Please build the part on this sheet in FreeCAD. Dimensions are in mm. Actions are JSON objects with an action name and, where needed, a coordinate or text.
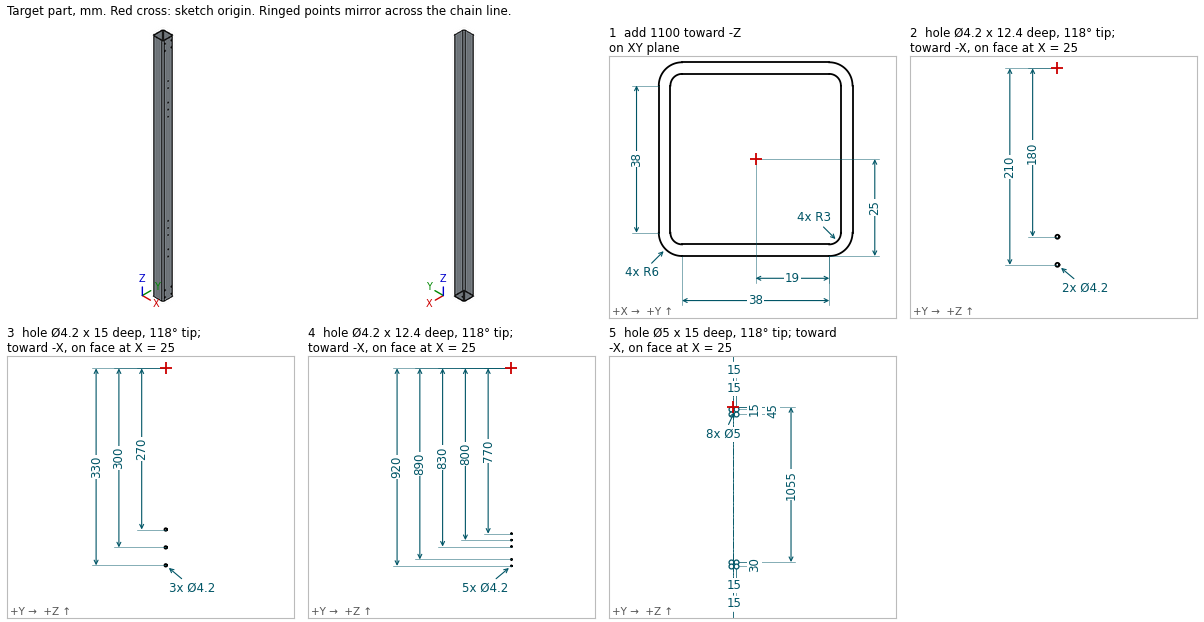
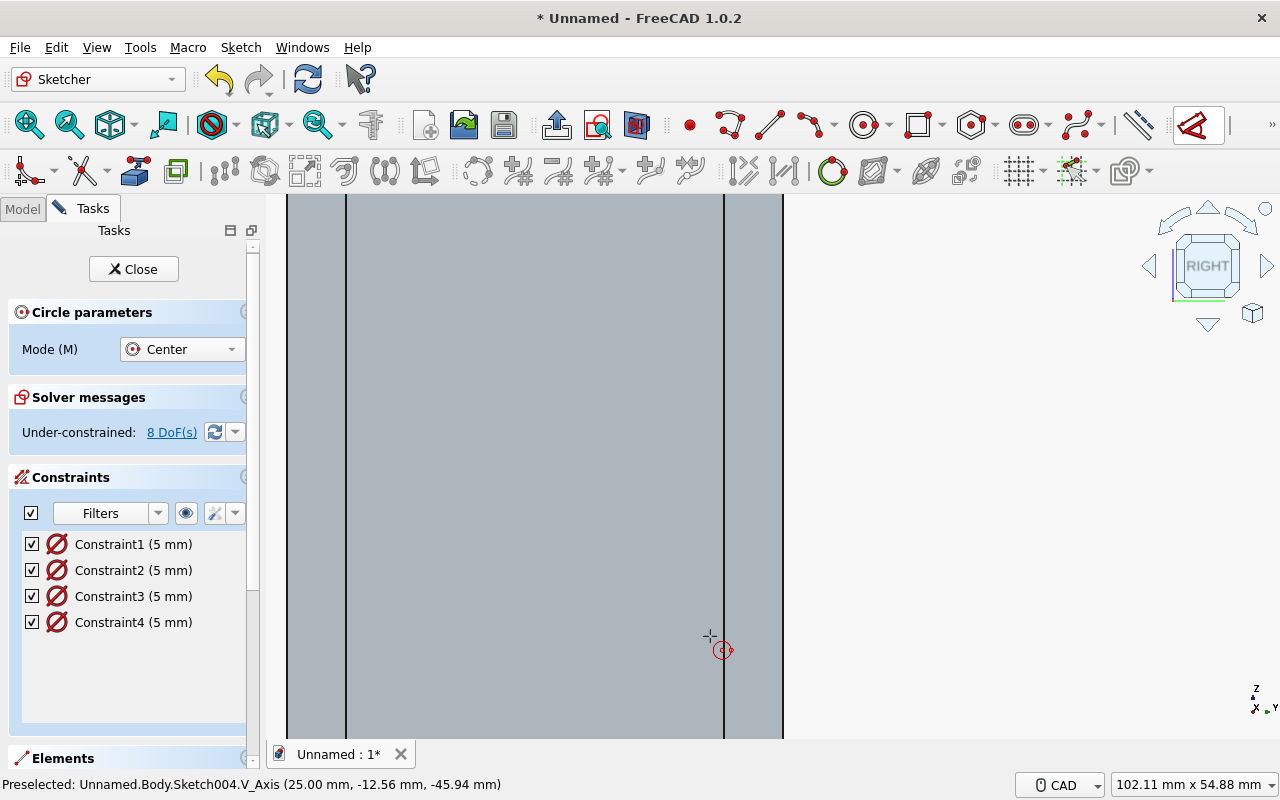
{"action": "scroll", "coordinate": [710, 637], "scroll_direction": "down", "scroll_amount": 17}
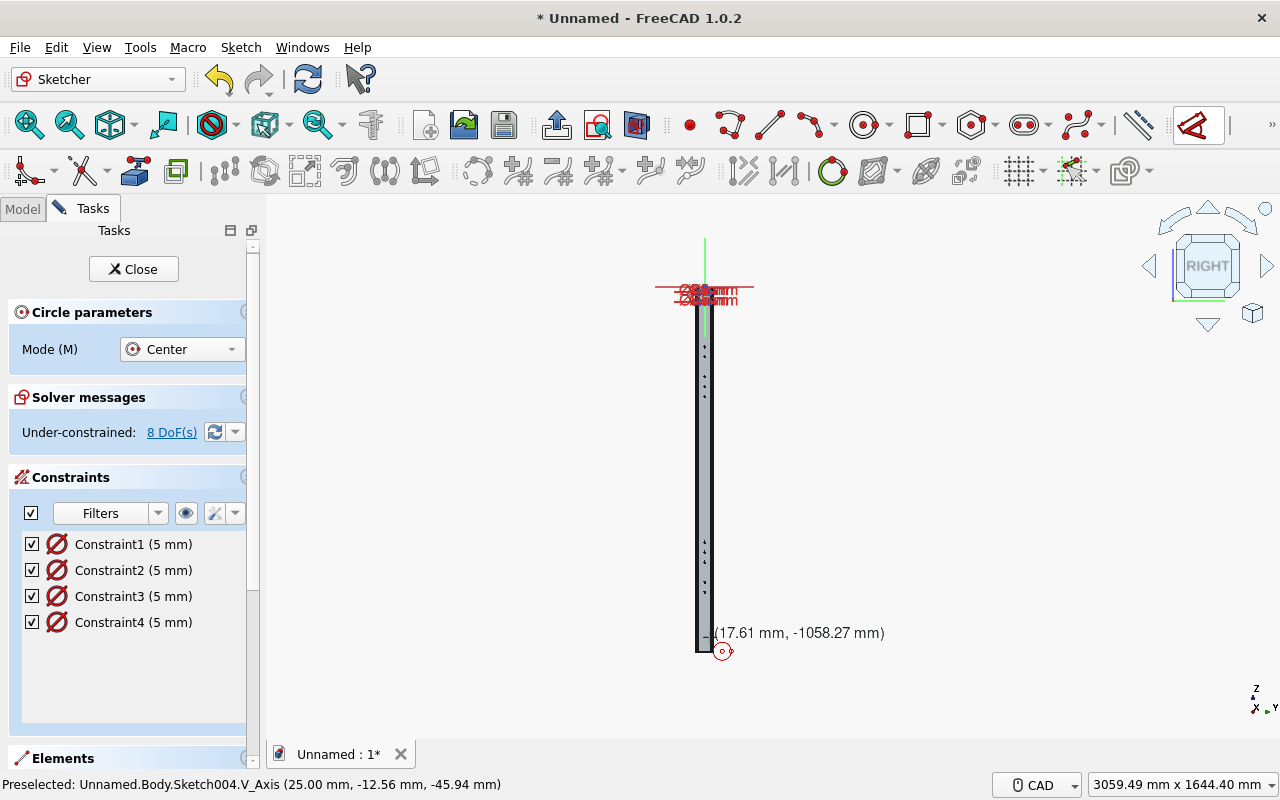
{"action": "scroll", "coordinate": [710, 637], "scroll_direction": "up", "scroll_amount": 6}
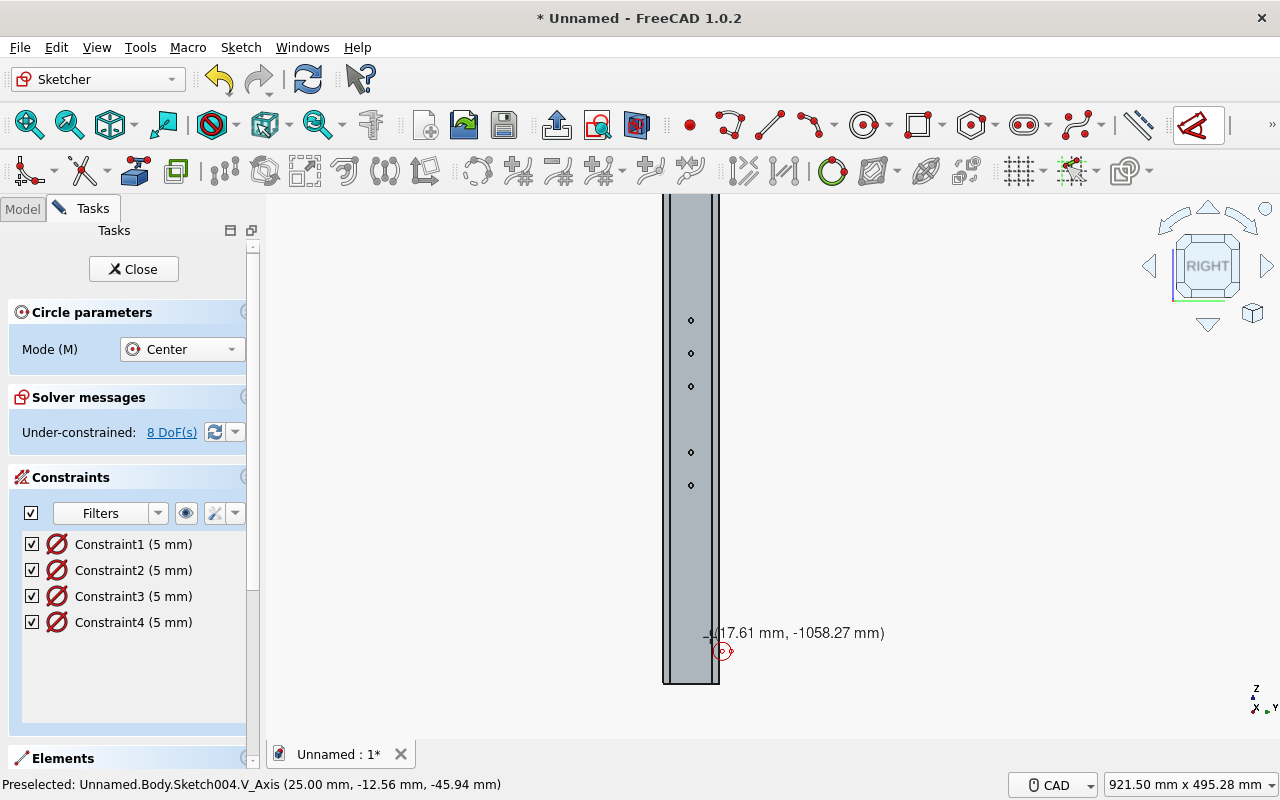
{"action": "left_click", "coordinate": [708, 634]}
{"action": "mouse_move", "coordinate": [709, 632]}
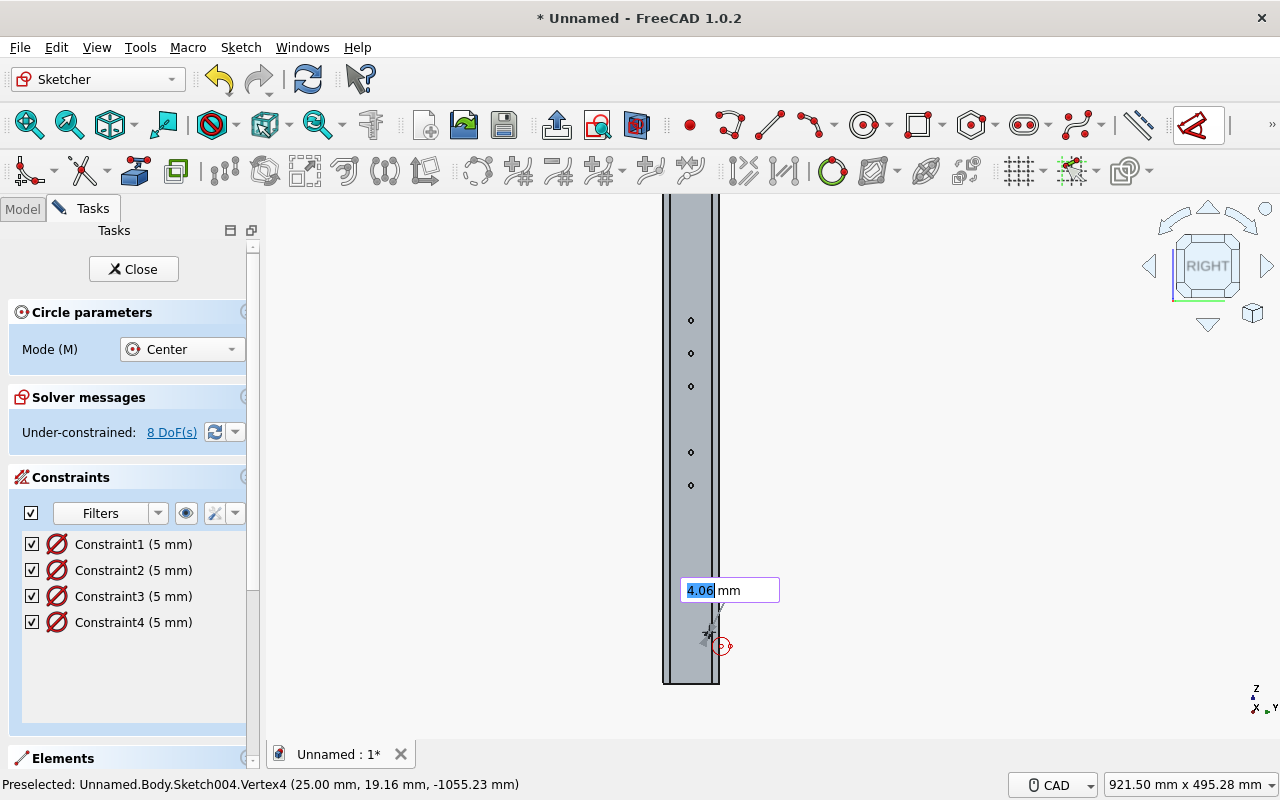
{"action": "type", "text": "5"}
{"action": "key", "text": "Return"}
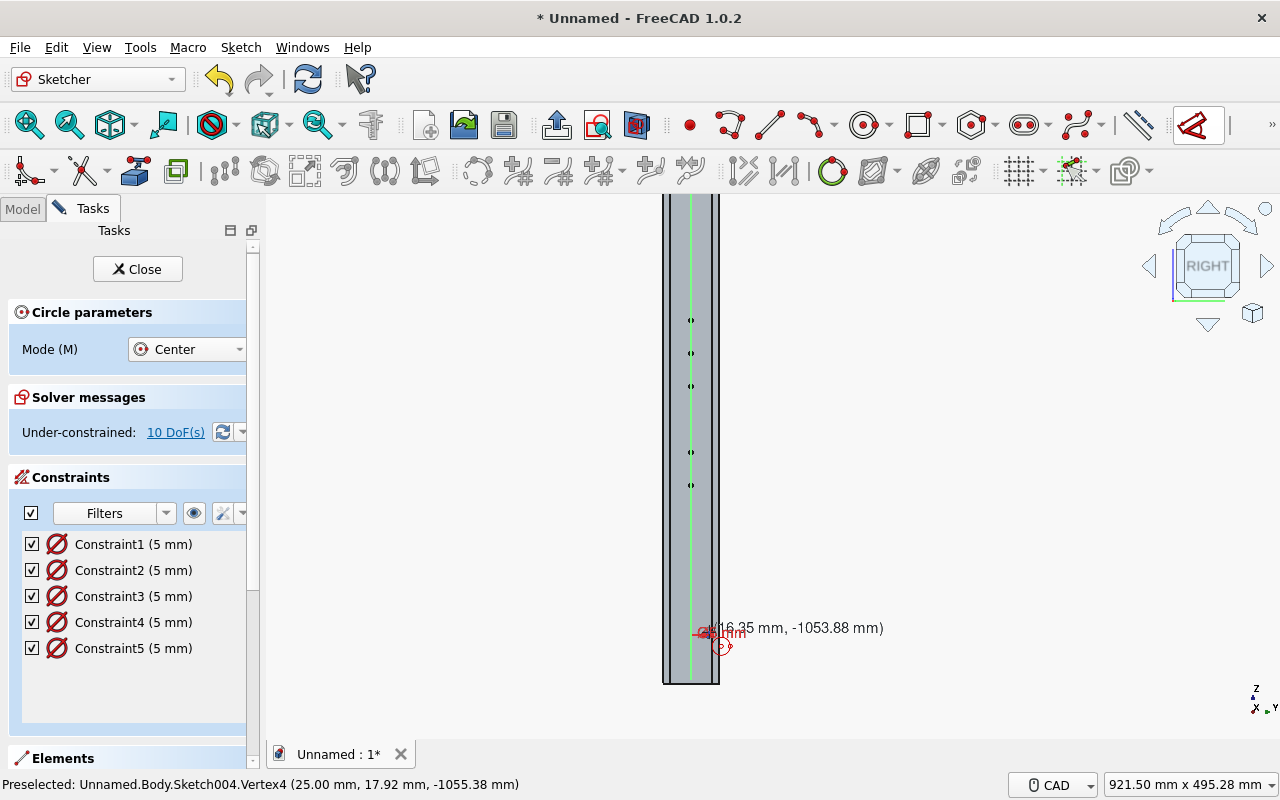
{"action": "scroll", "coordinate": [708, 667], "scroll_direction": "up", "scroll_amount": 11}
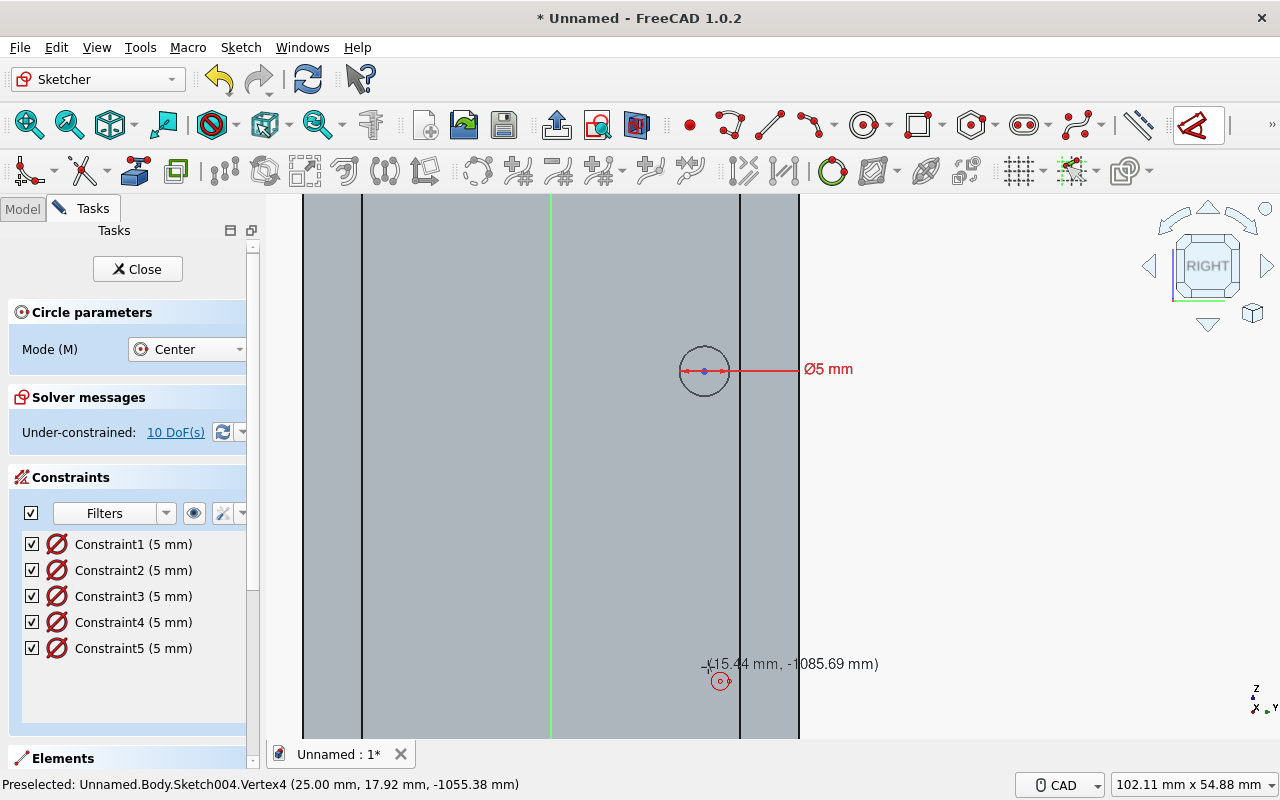
{"action": "scroll", "coordinate": [710, 645], "scroll_direction": "down", "scroll_amount": 17}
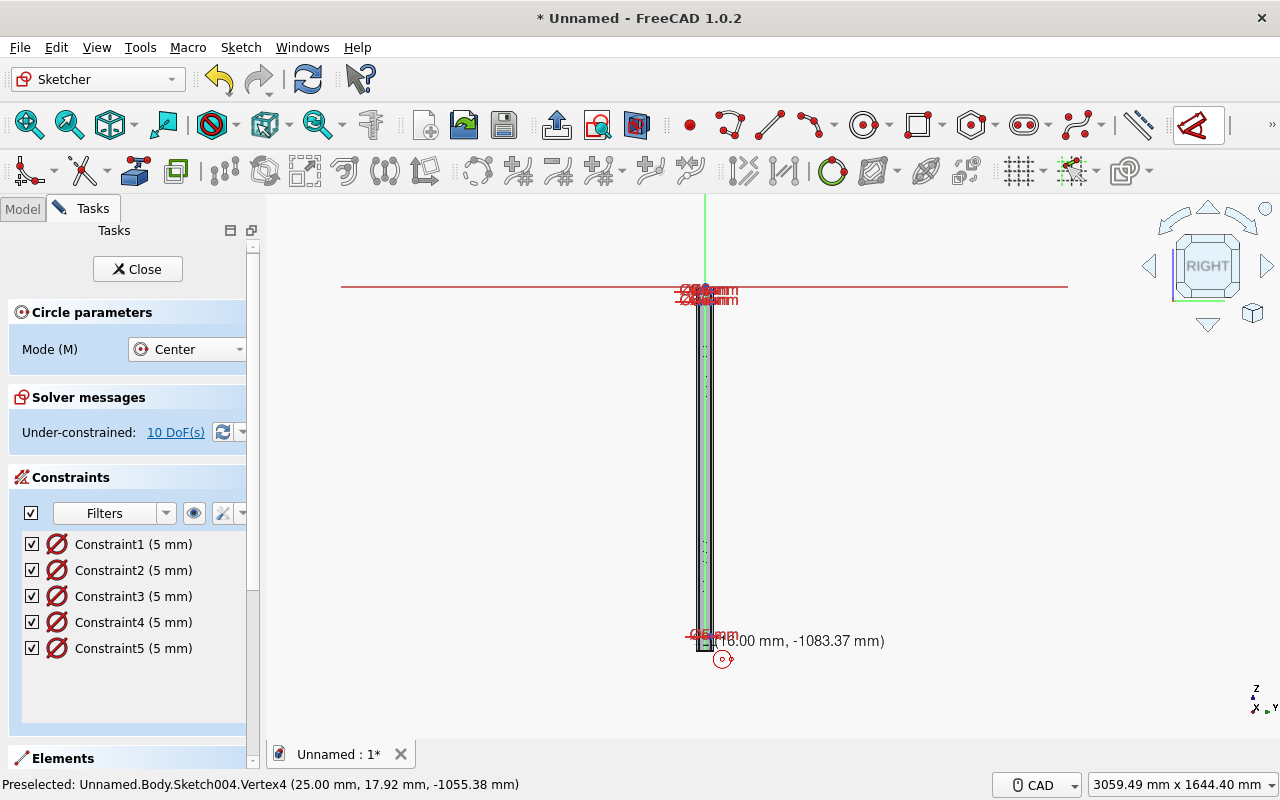
{"action": "scroll", "coordinate": [710, 646], "scroll_direction": "up", "scroll_amount": 6}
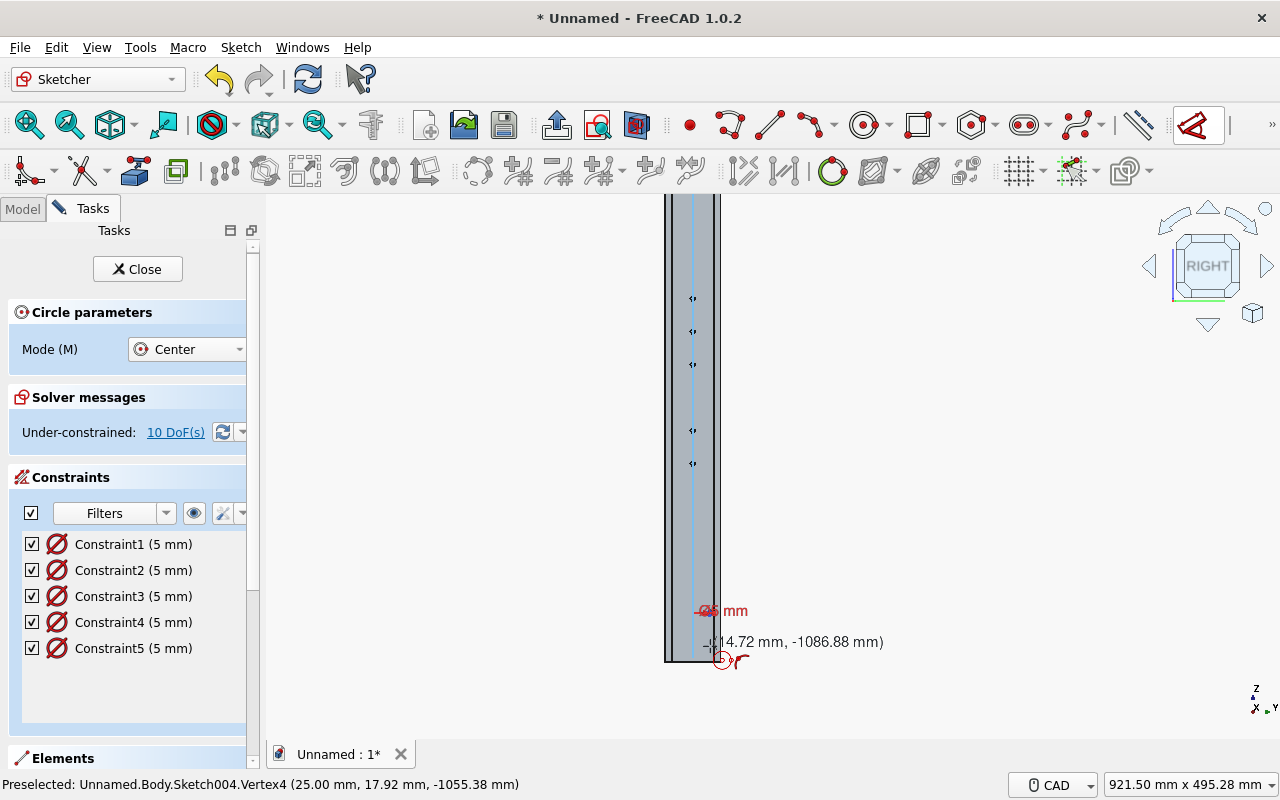
{"action": "left_click", "coordinate": [709, 645]}
{"action": "mouse_move", "coordinate": [711, 643]}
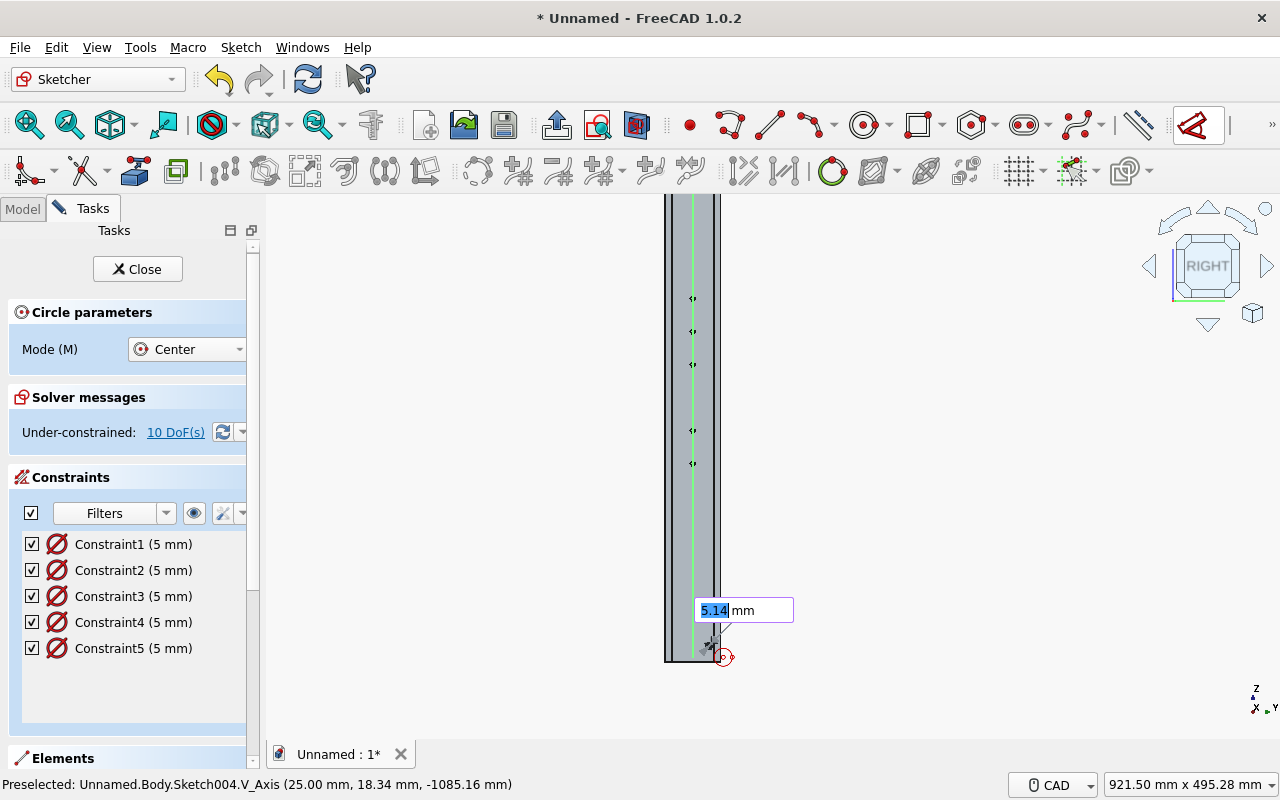
{"action": "type", "text": "5"}
{"action": "key", "text": "Return"}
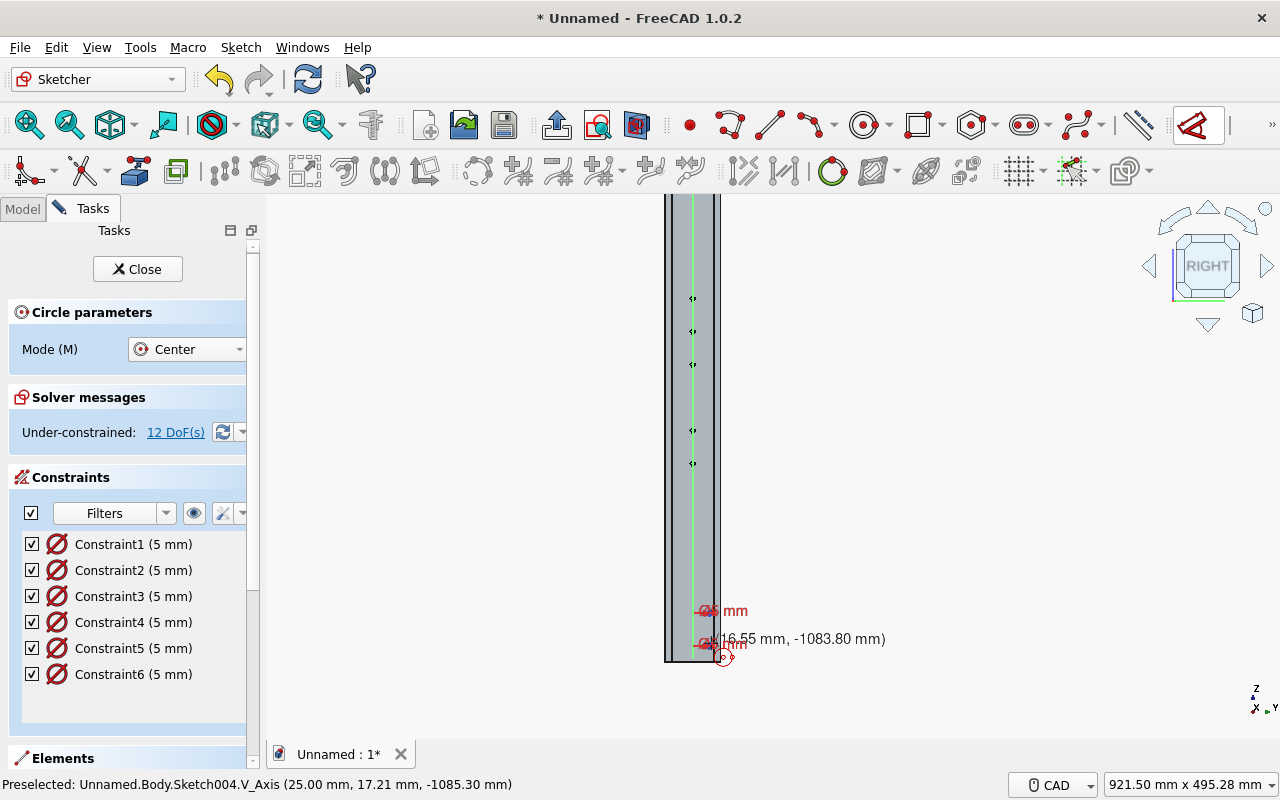
{"action": "scroll", "coordinate": [676, 612], "scroll_direction": "up", "scroll_amount": 11}